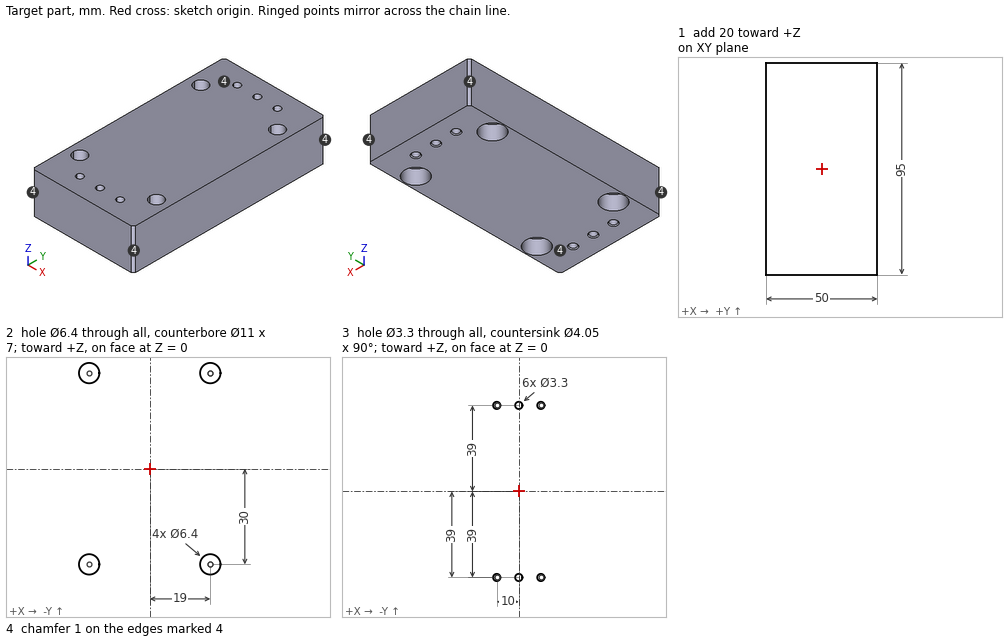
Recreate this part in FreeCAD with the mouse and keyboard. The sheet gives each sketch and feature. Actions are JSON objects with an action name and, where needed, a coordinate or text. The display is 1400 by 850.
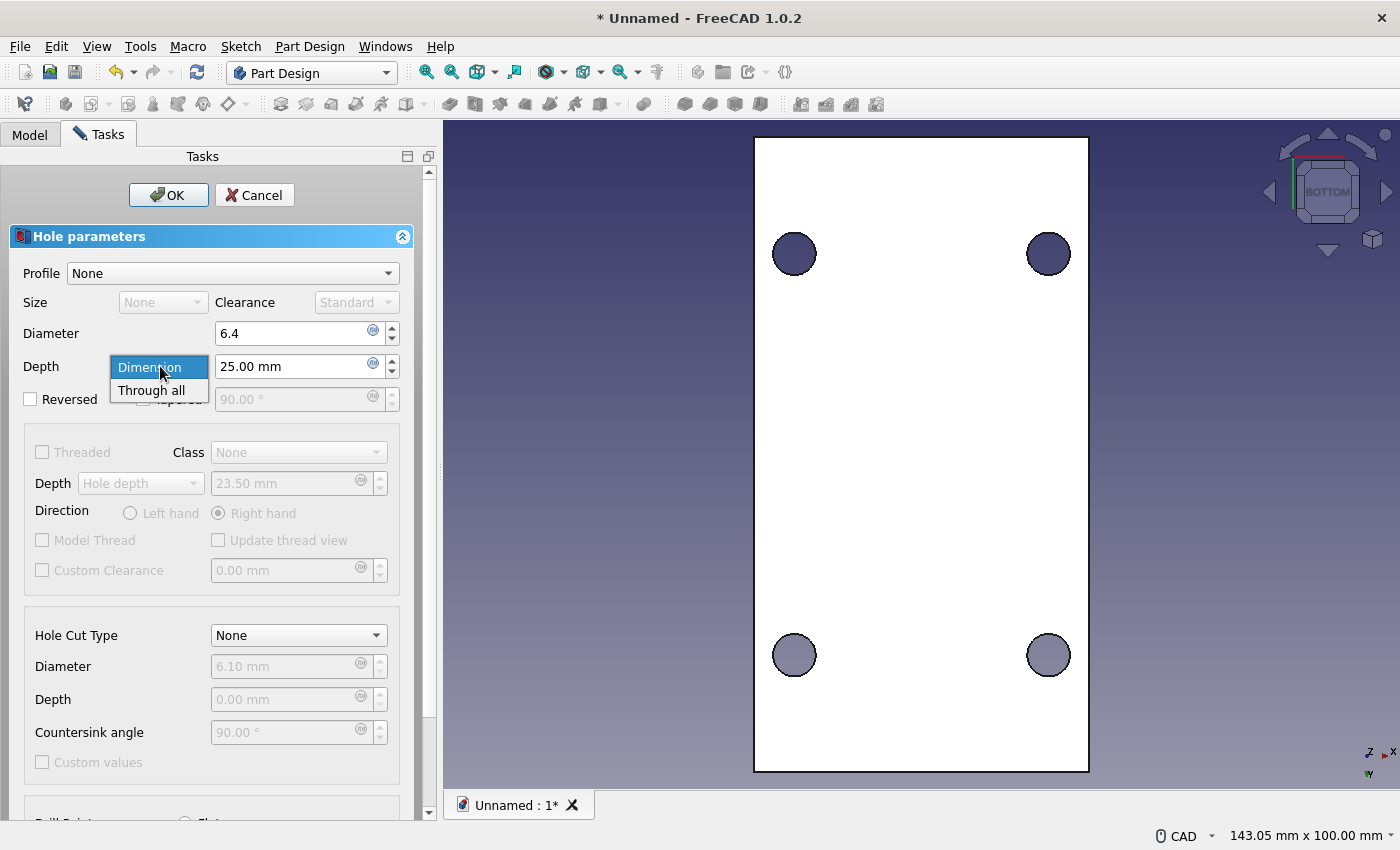
{"action": "left_click", "coordinate": [158, 390]}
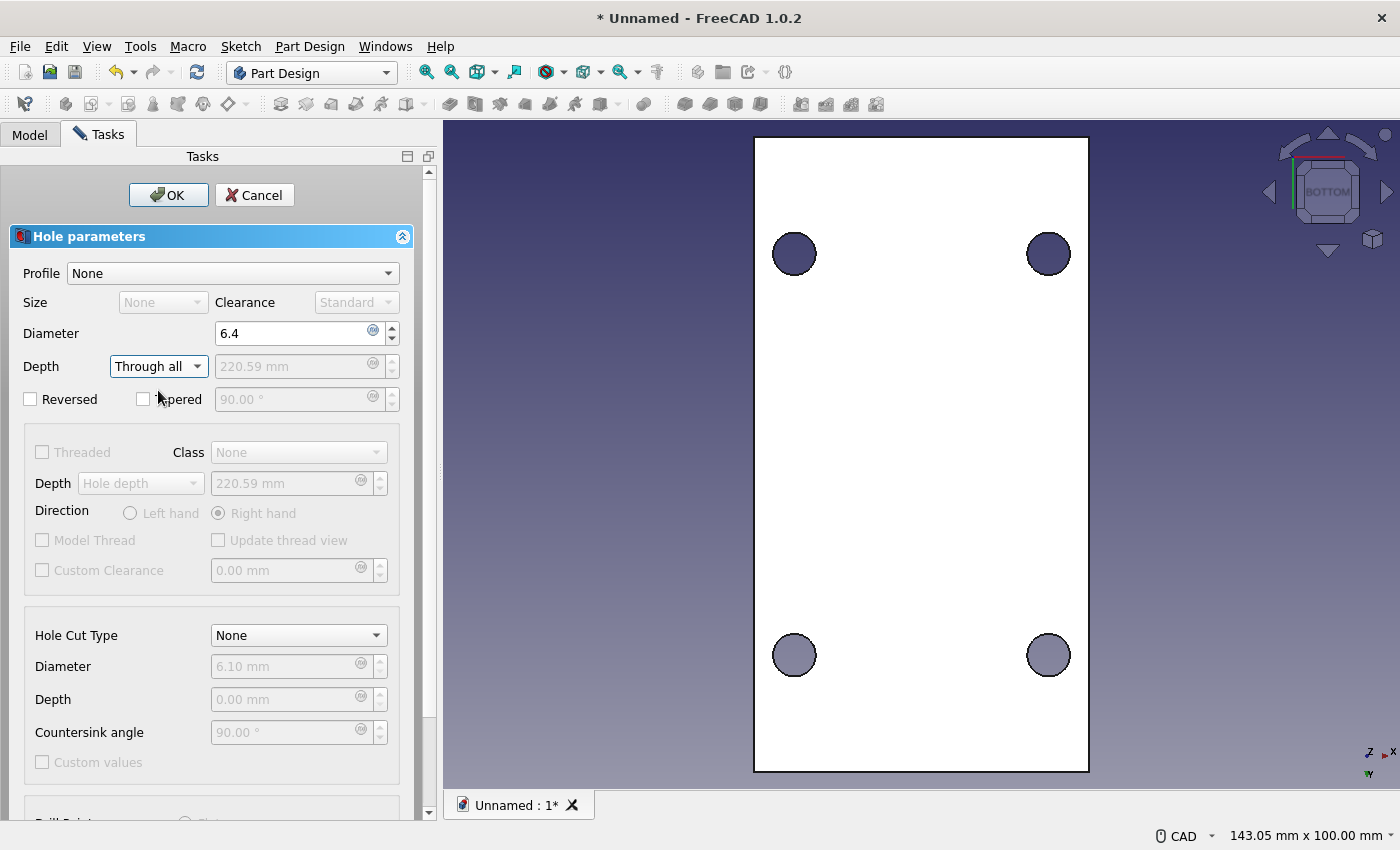
{"action": "left_click", "coordinate": [300, 636]}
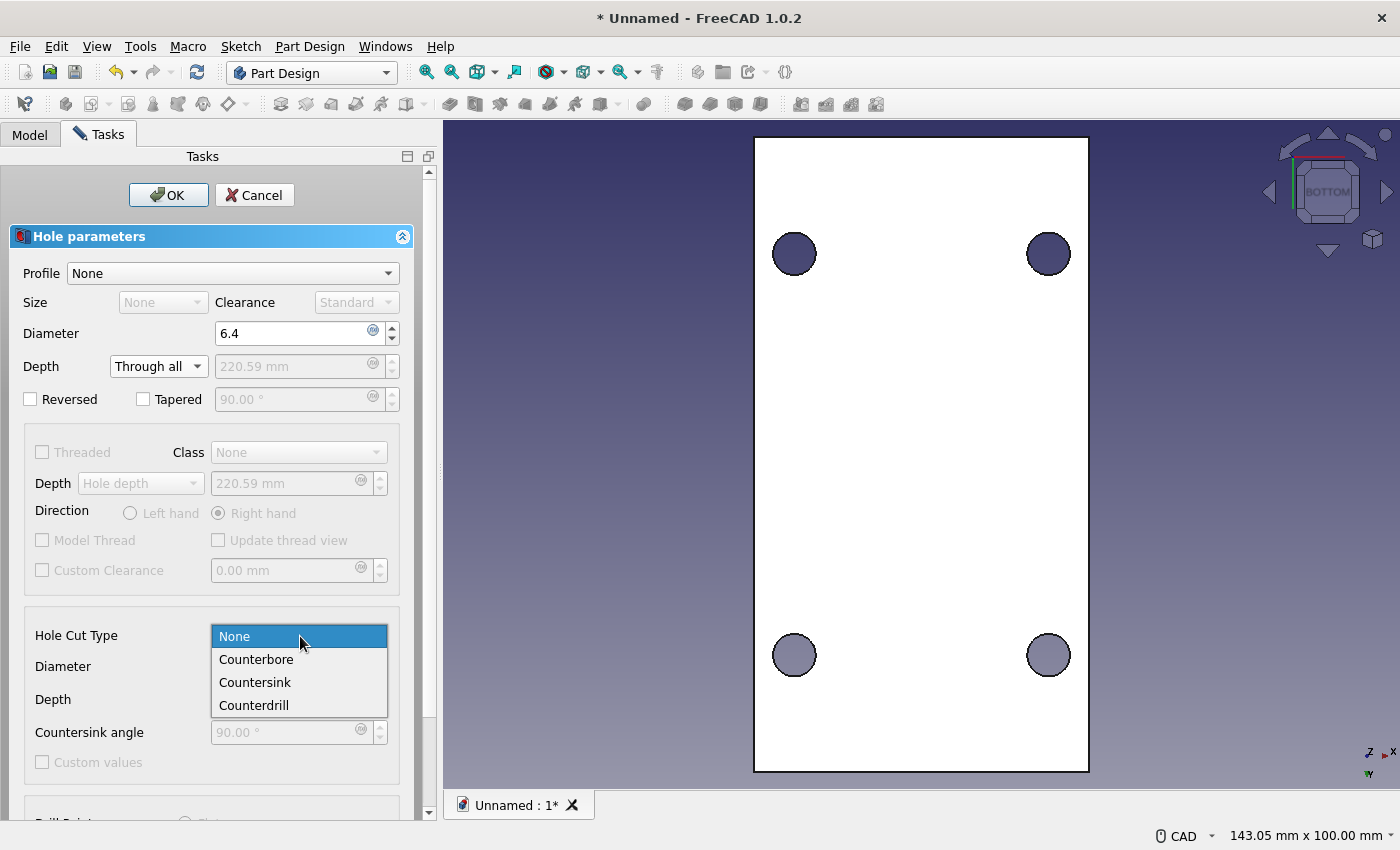
{"action": "left_click", "coordinate": [298, 660]}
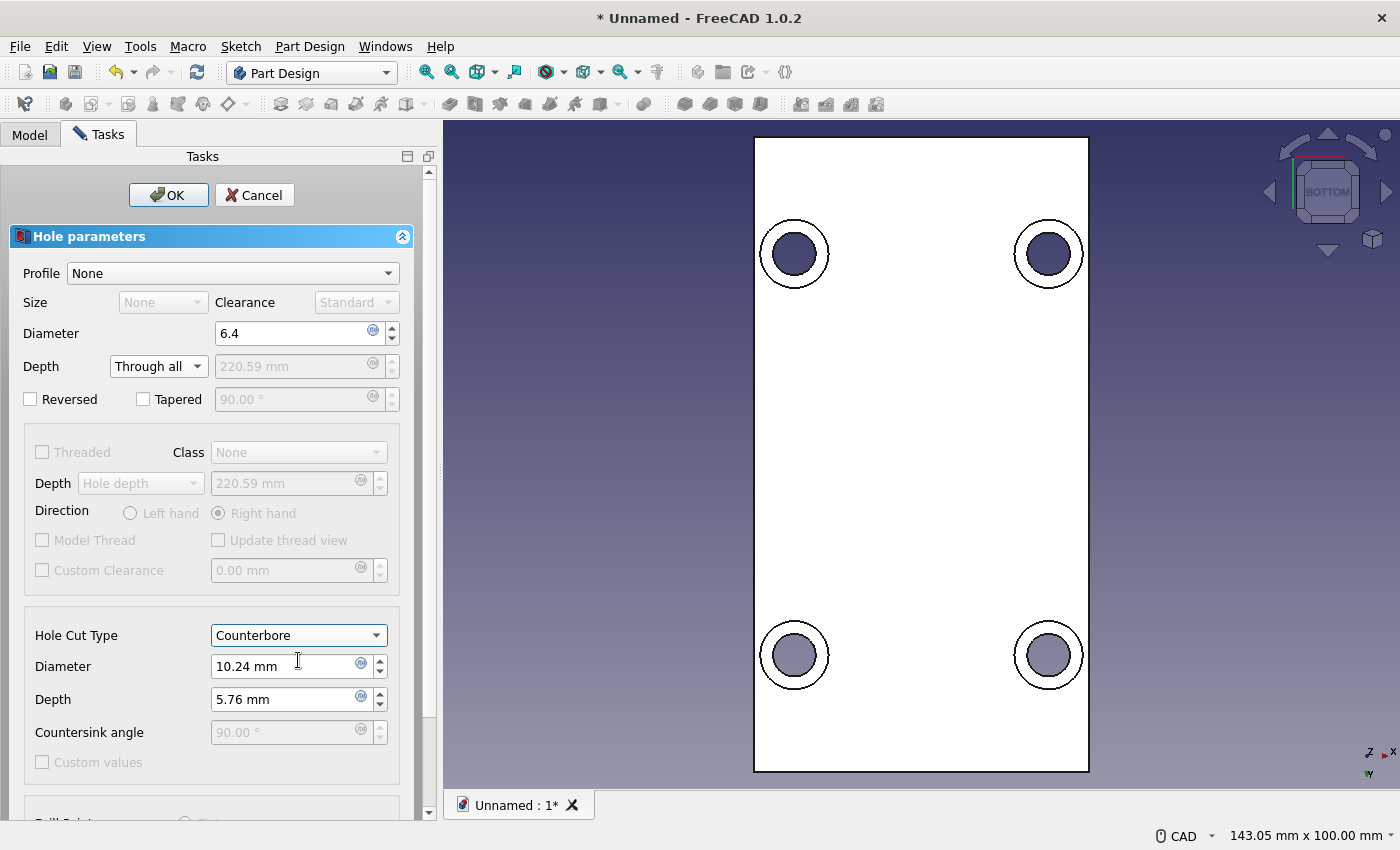
{"action": "triple_click", "coordinate": [292, 666]}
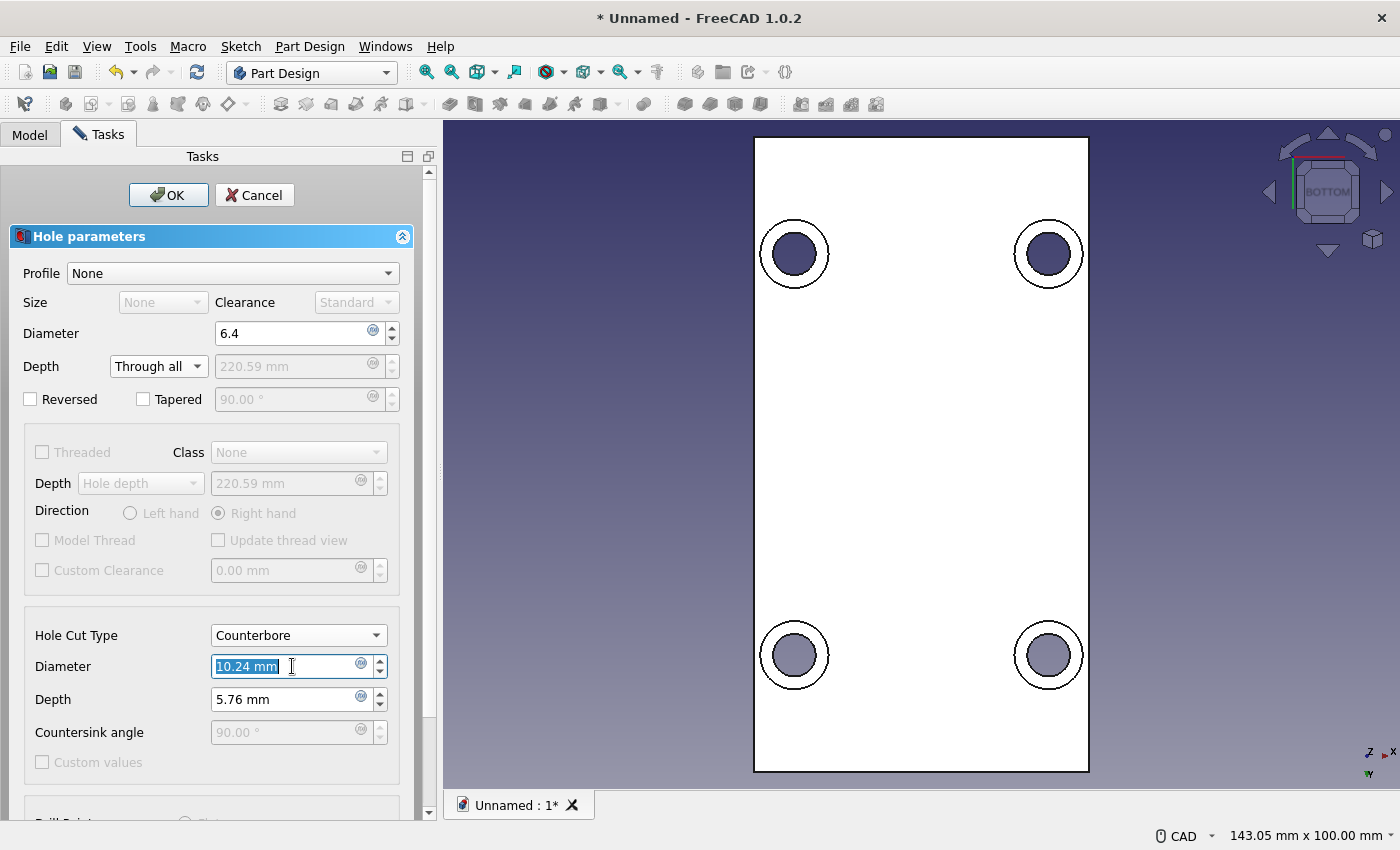
{"action": "type", "text": "11"}
{"action": "key", "text": "Tab"}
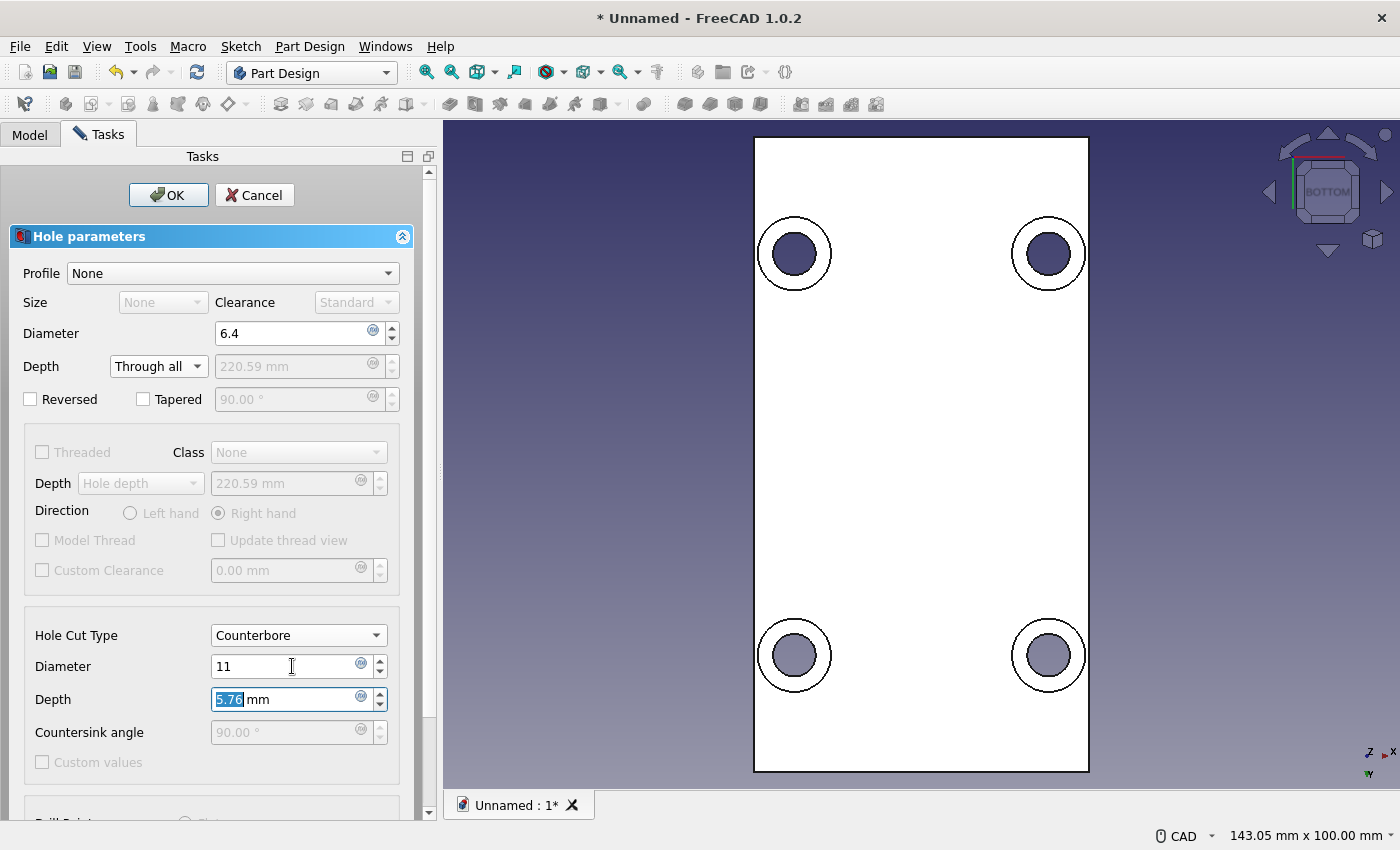
{"action": "type", "text": "7"}
{"action": "key", "text": "Tab"}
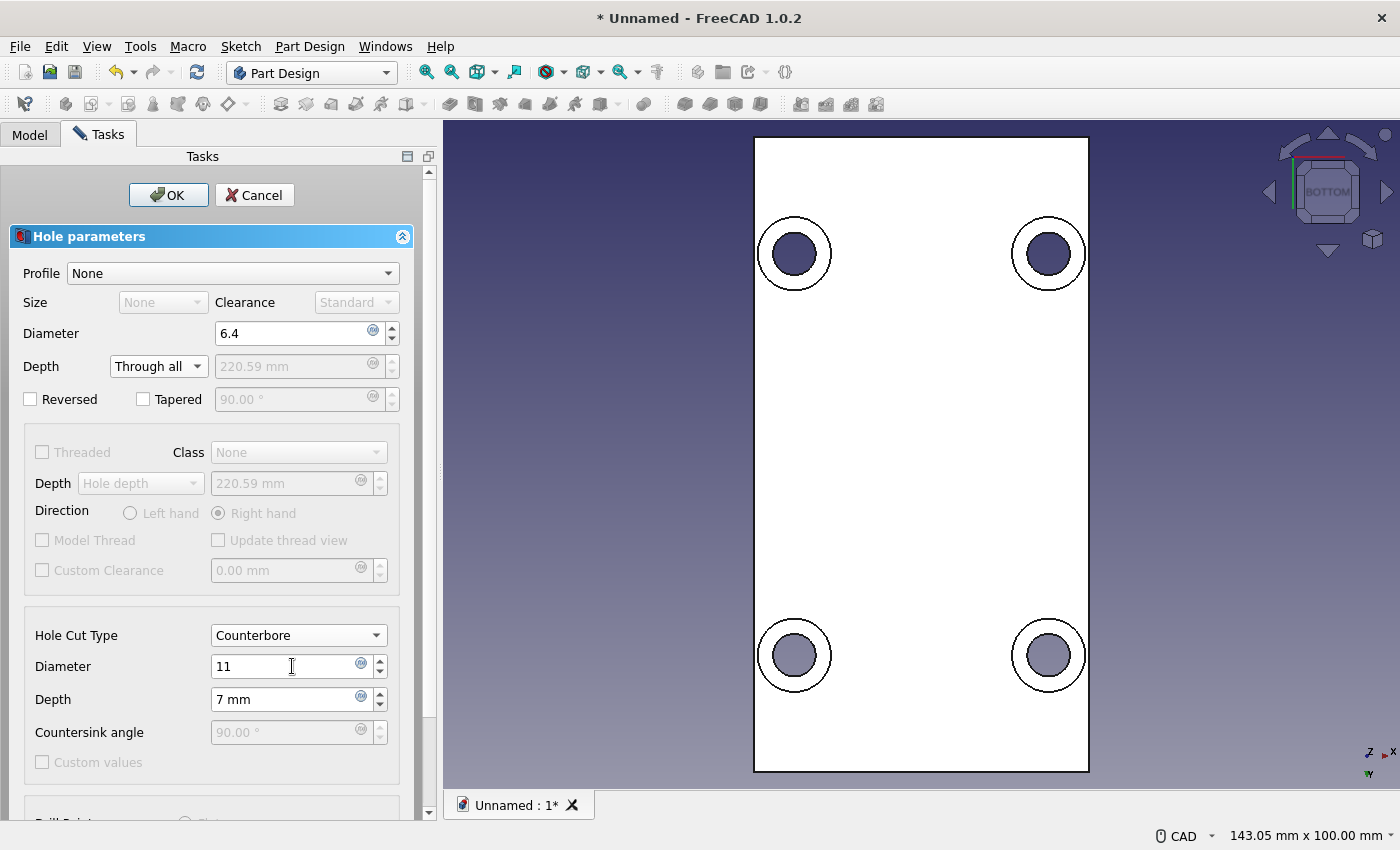
{"action": "left_click", "coordinate": [169, 195]}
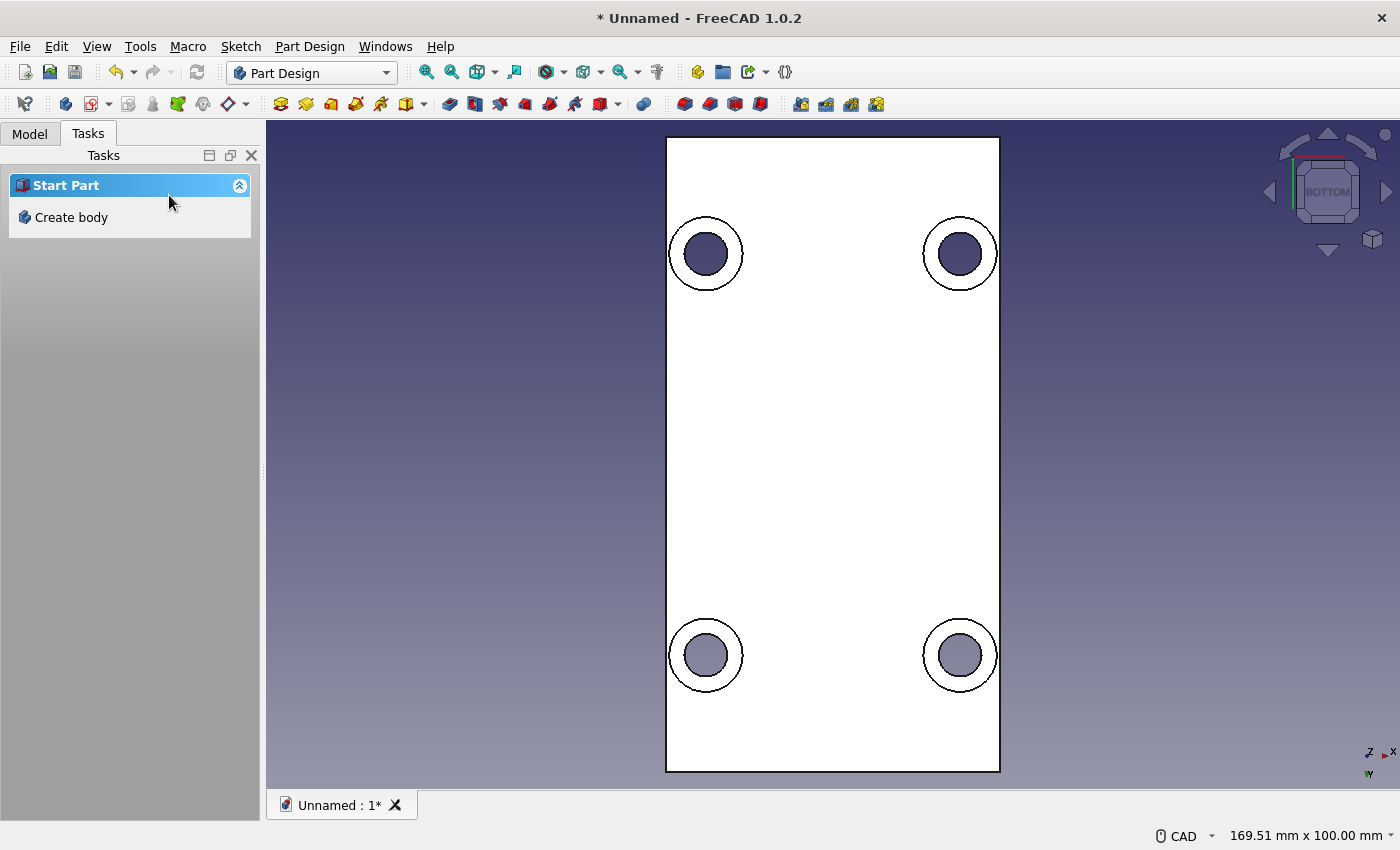
{"action": "left_click", "coordinate": [833, 454]}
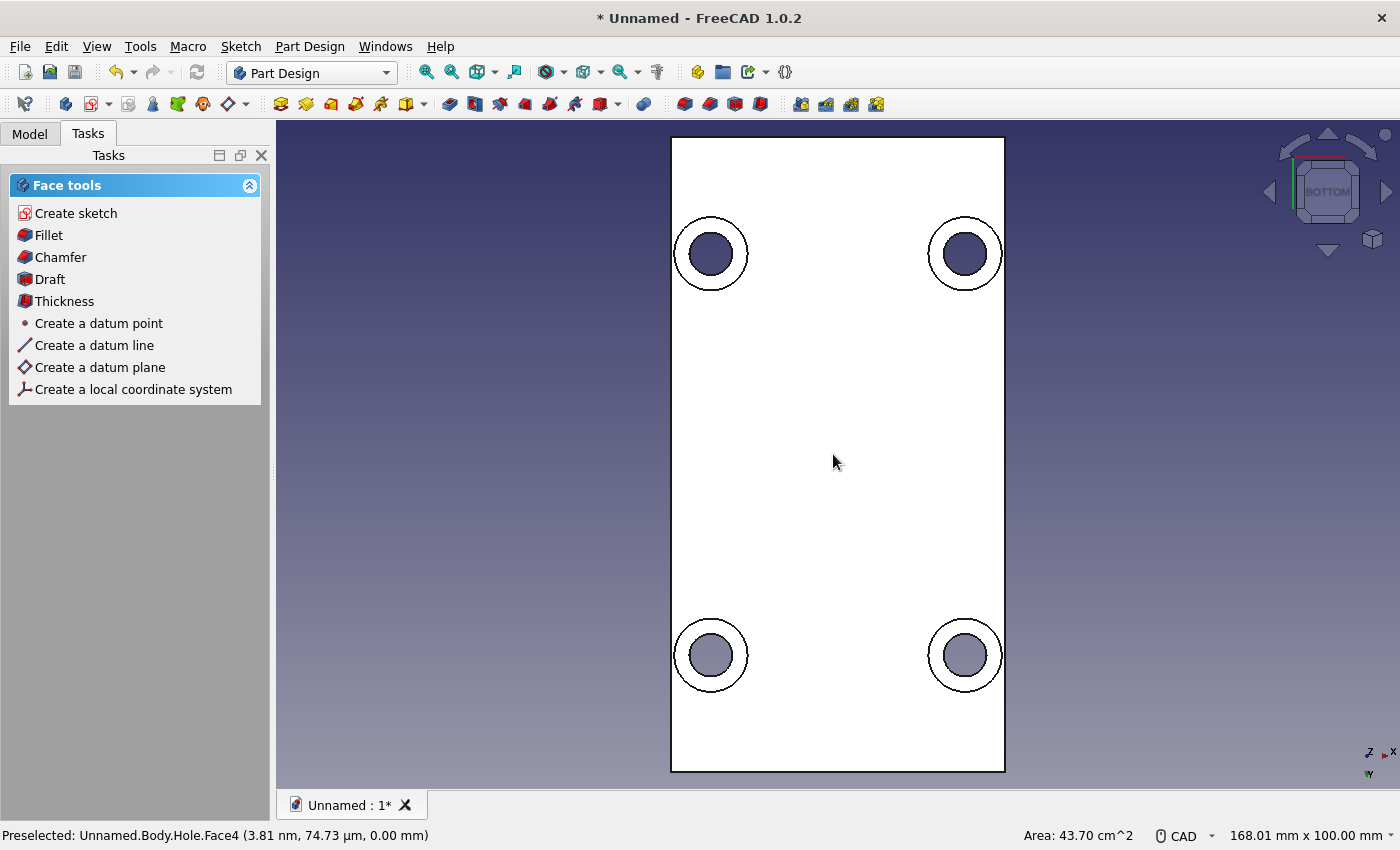
{"action": "left_click", "coordinate": [90, 104]}